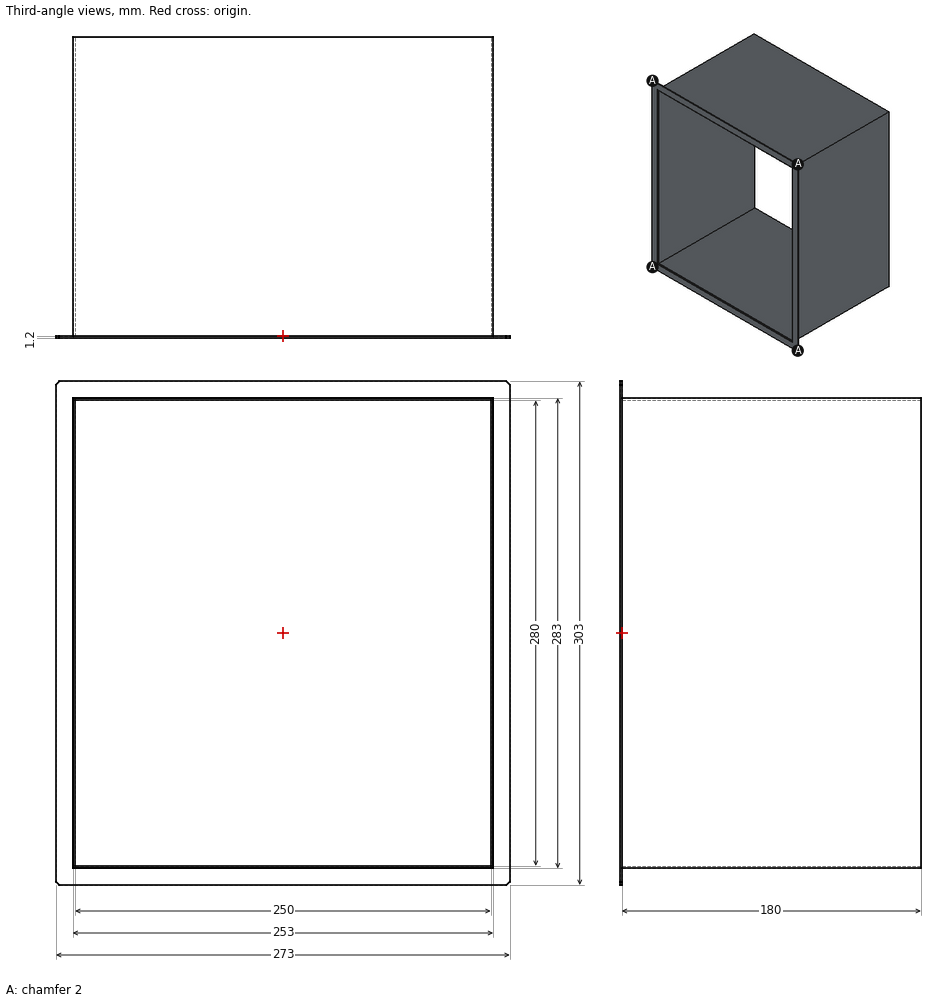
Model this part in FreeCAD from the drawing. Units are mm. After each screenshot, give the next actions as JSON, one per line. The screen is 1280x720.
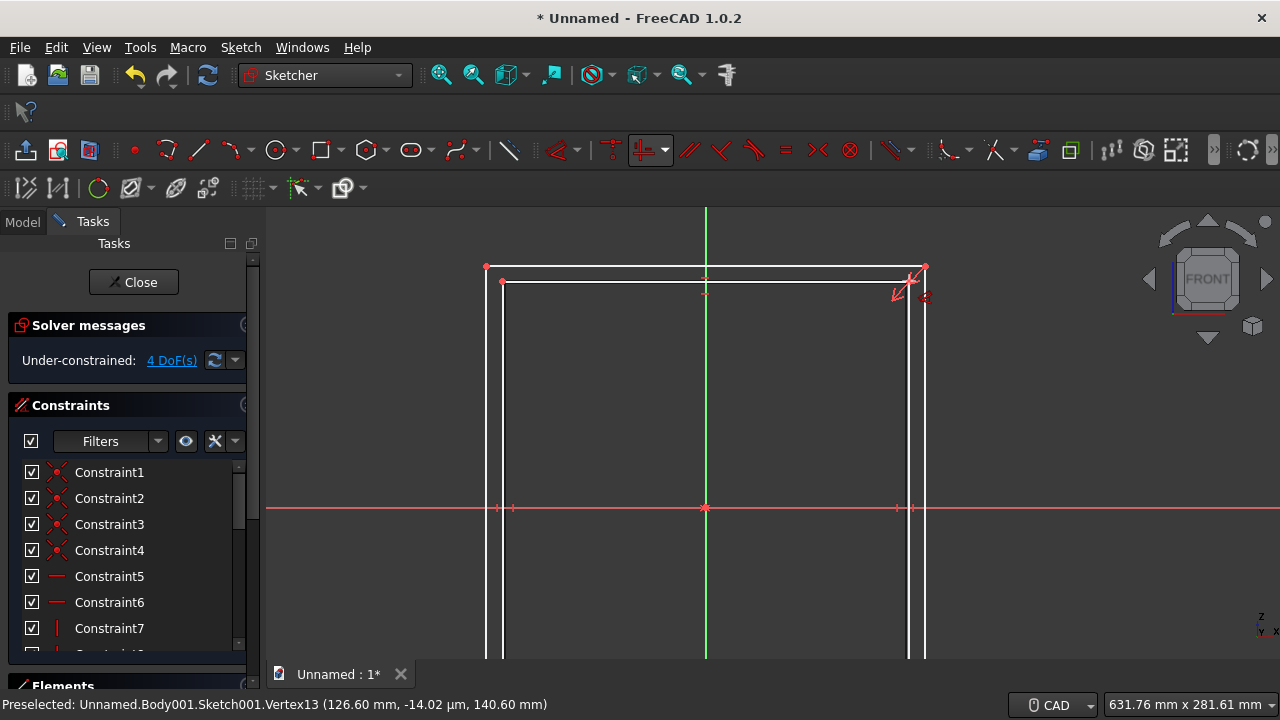
{"action": "scroll", "coordinate": [703, 342], "scroll_direction": "down", "scroll_amount": 3}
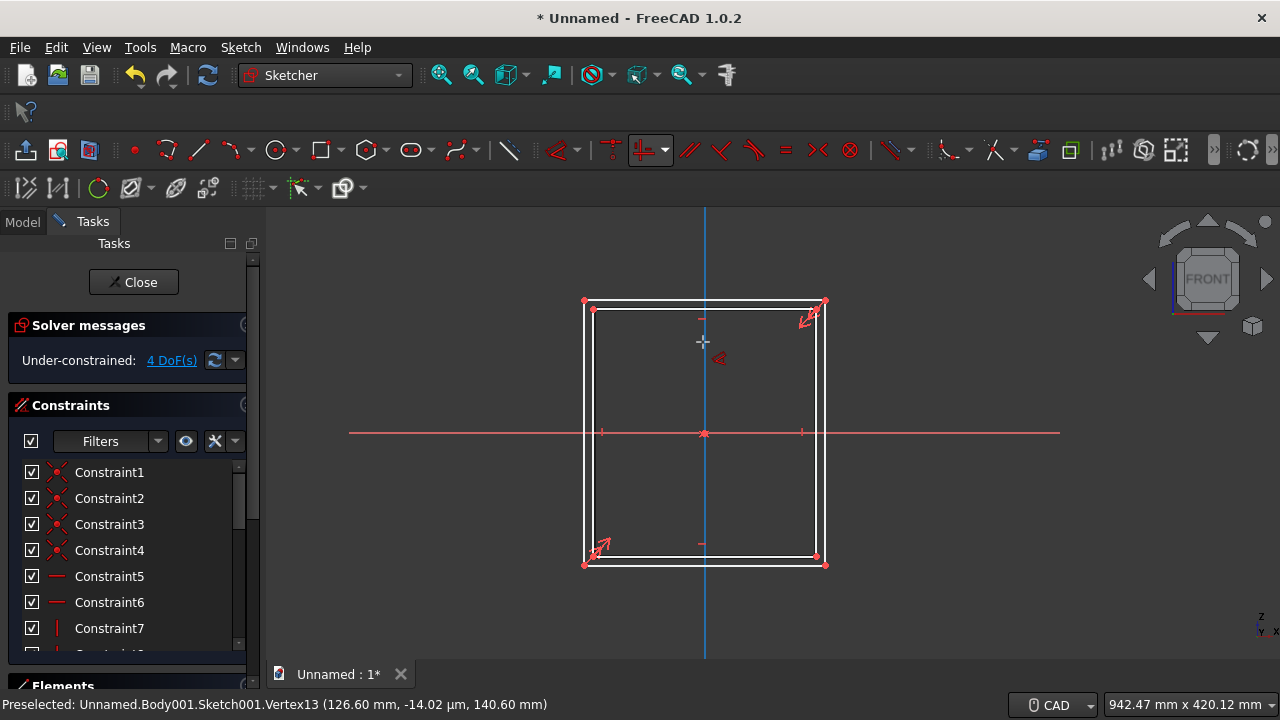
{"action": "scroll", "coordinate": [657, 566], "scroll_direction": "up", "scroll_amount": 3}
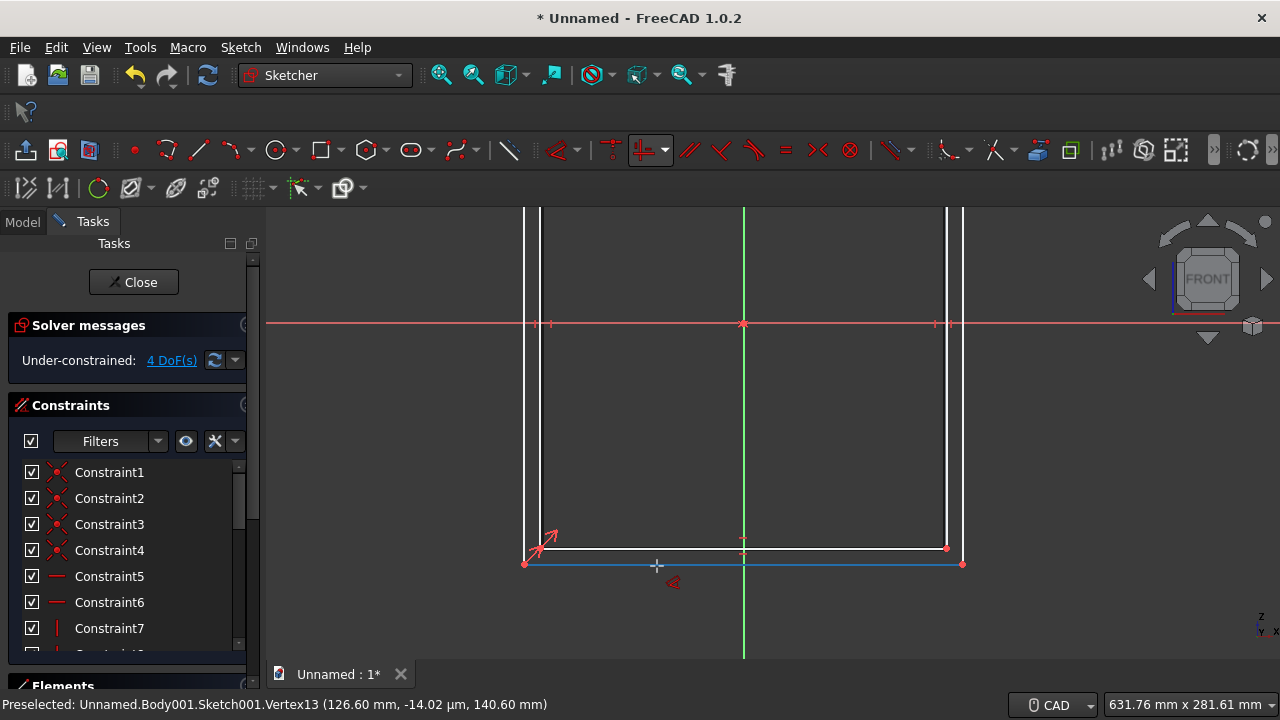
{"action": "left_click", "coordinate": [656, 565]}
{"action": "left_click", "coordinate": [643, 599]}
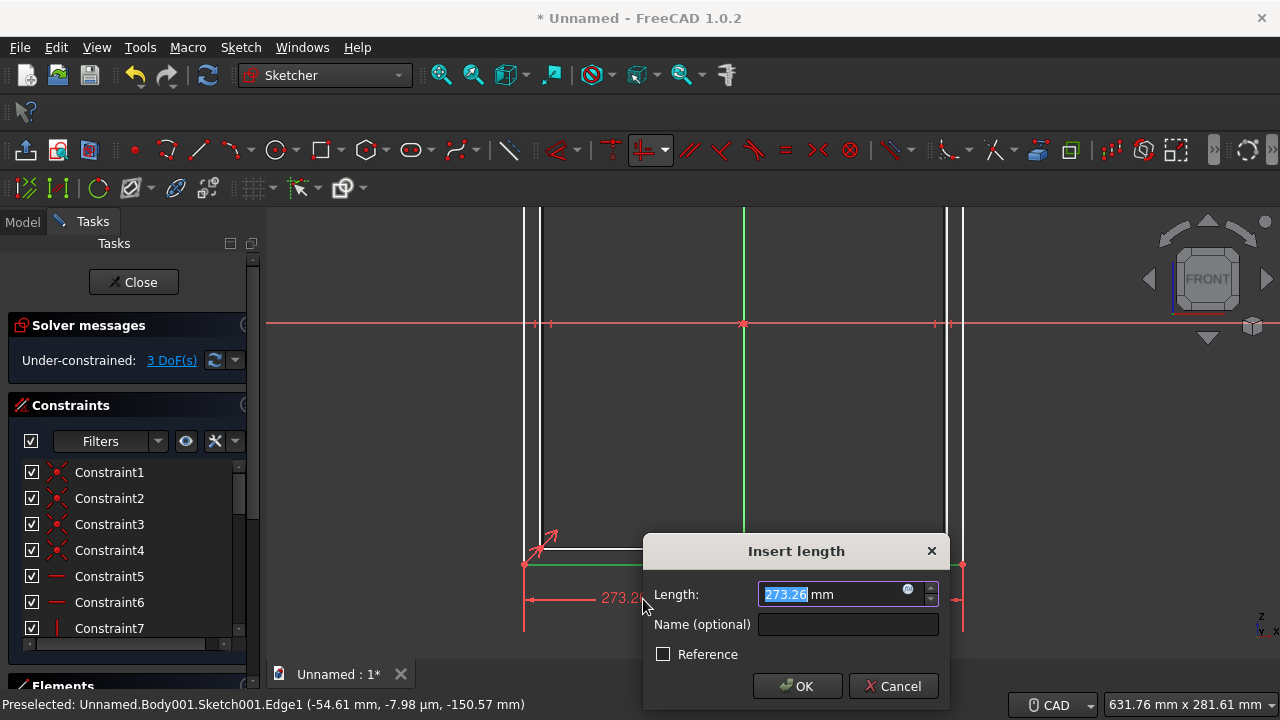
{"action": "type", "text": "273"}
{"action": "key", "text": "Return"}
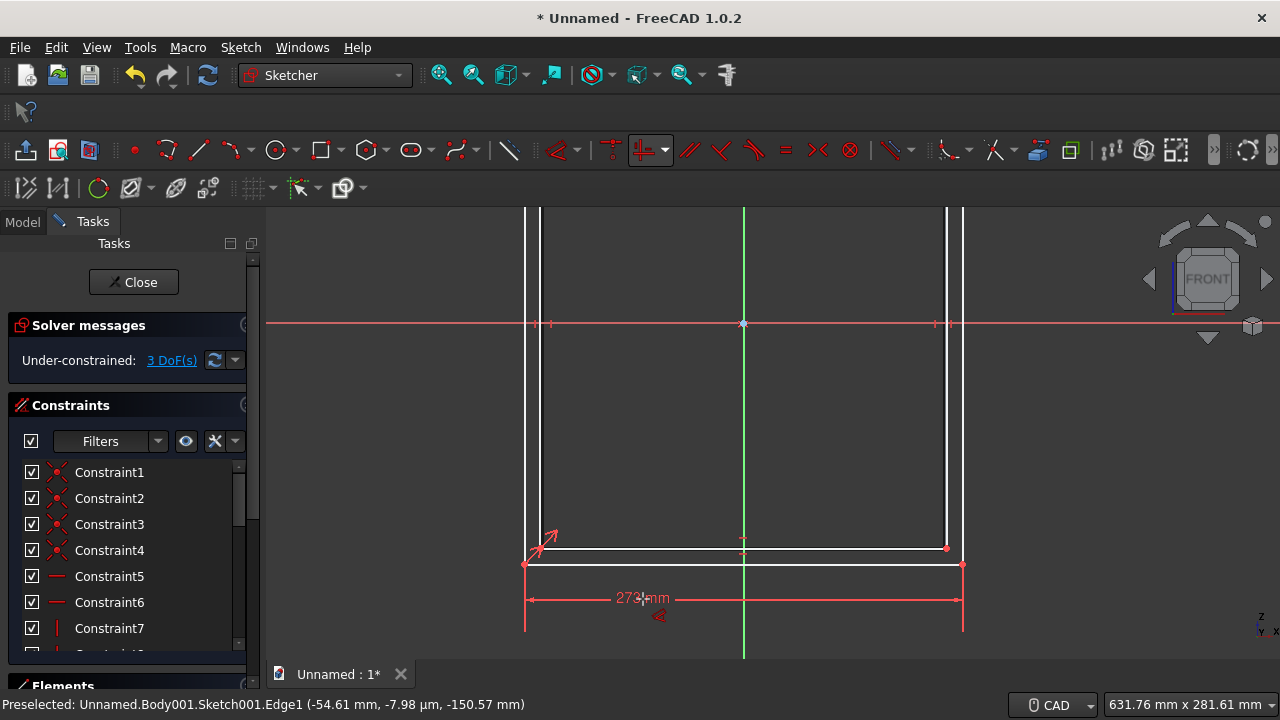
{"action": "left_click", "coordinate": [963, 420]}
{"action": "left_click", "coordinate": [997, 400]}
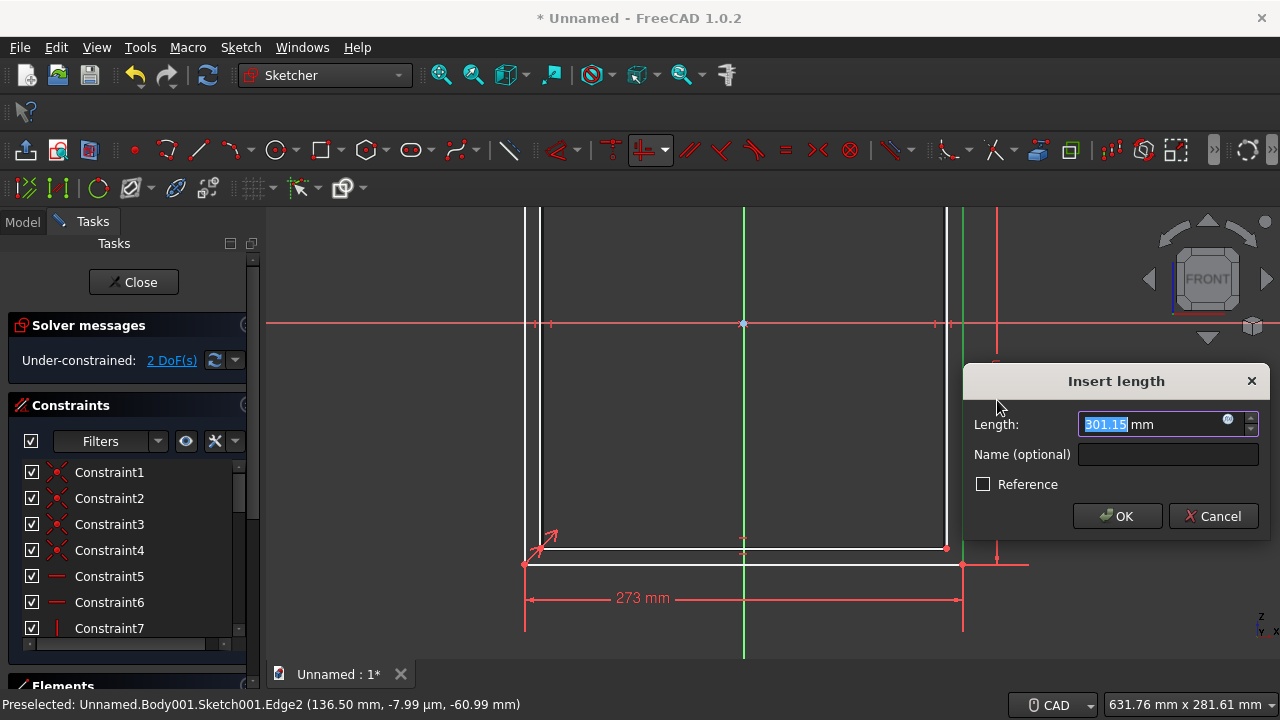
{"action": "type", "text": "303"}
{"action": "key", "text": "Return"}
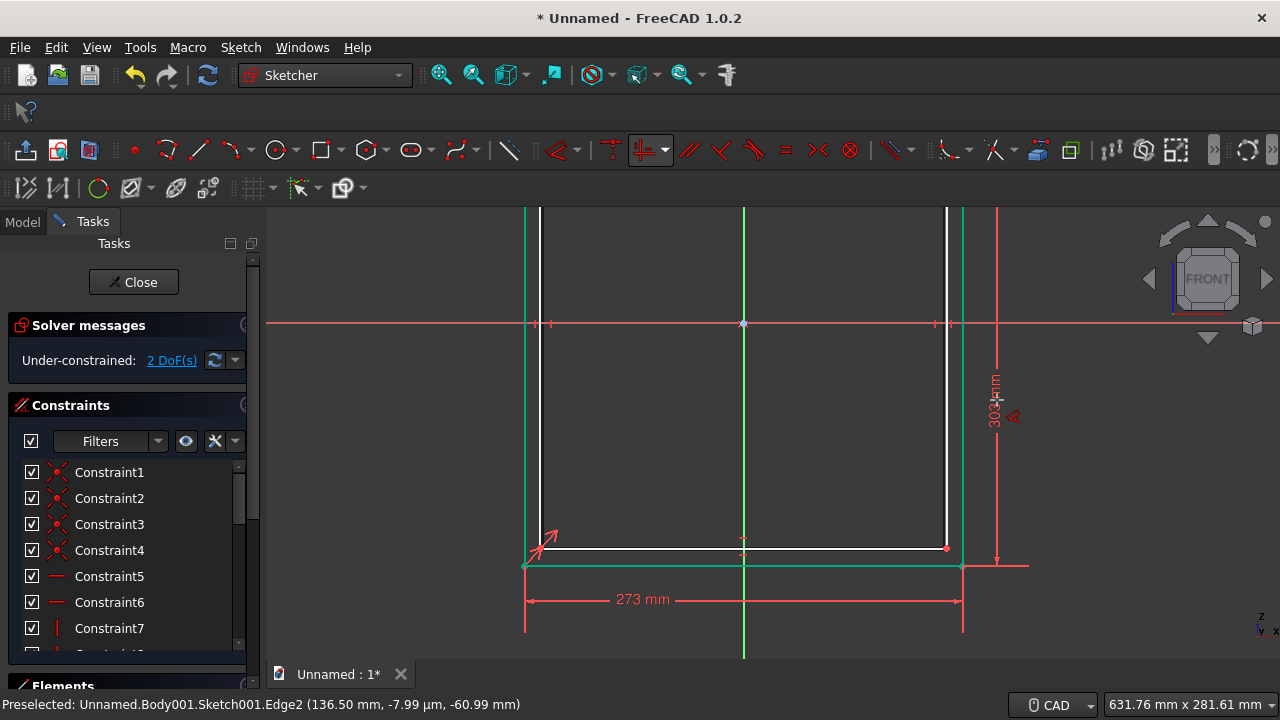
{"action": "left_click", "coordinate": [662, 549]}
{"action": "left_click", "coordinate": [837, 583]}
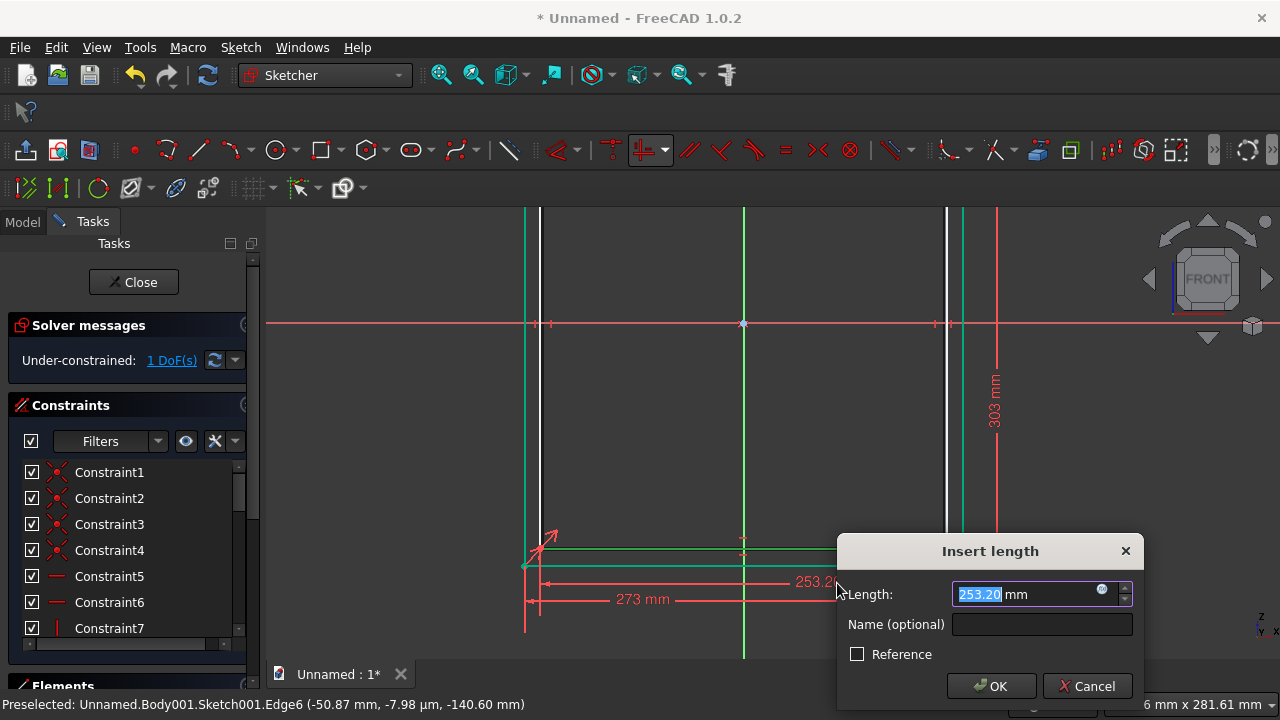
{"action": "type", "text": "253"}
{"action": "key", "text": "Return"}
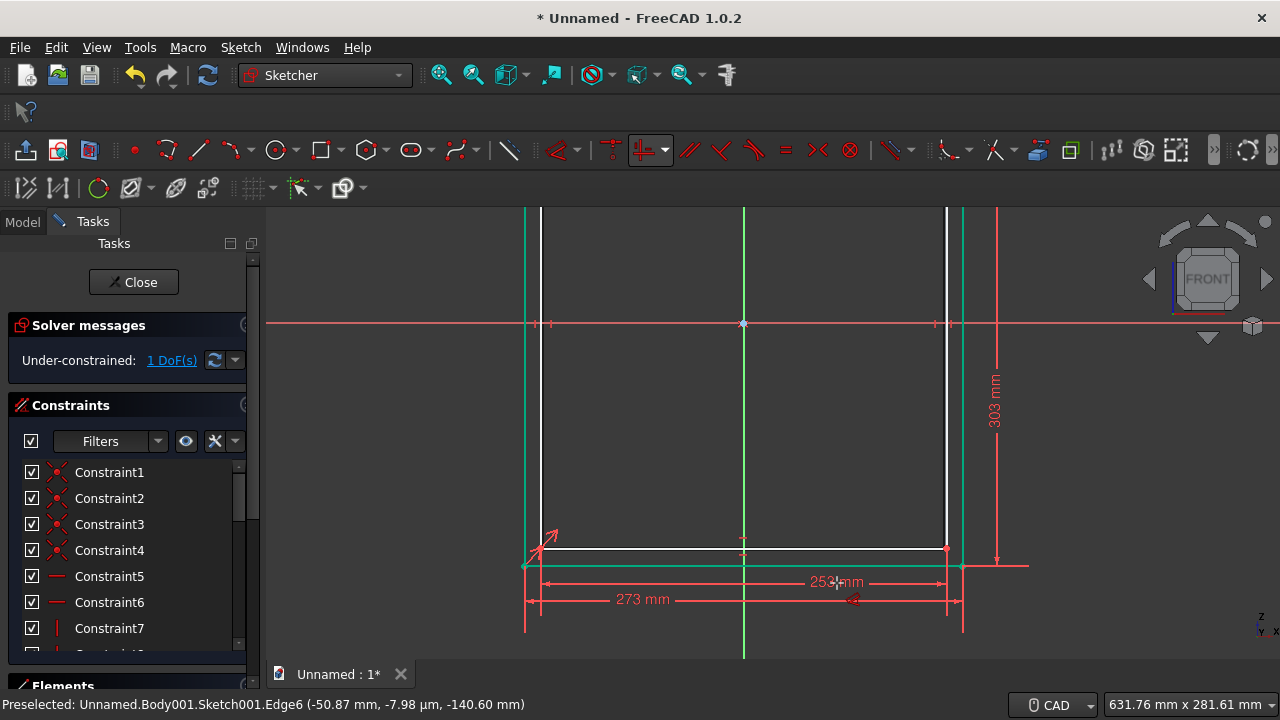
{"action": "left_click", "coordinate": [947, 413]}
{"action": "left_click", "coordinate": [981, 464]}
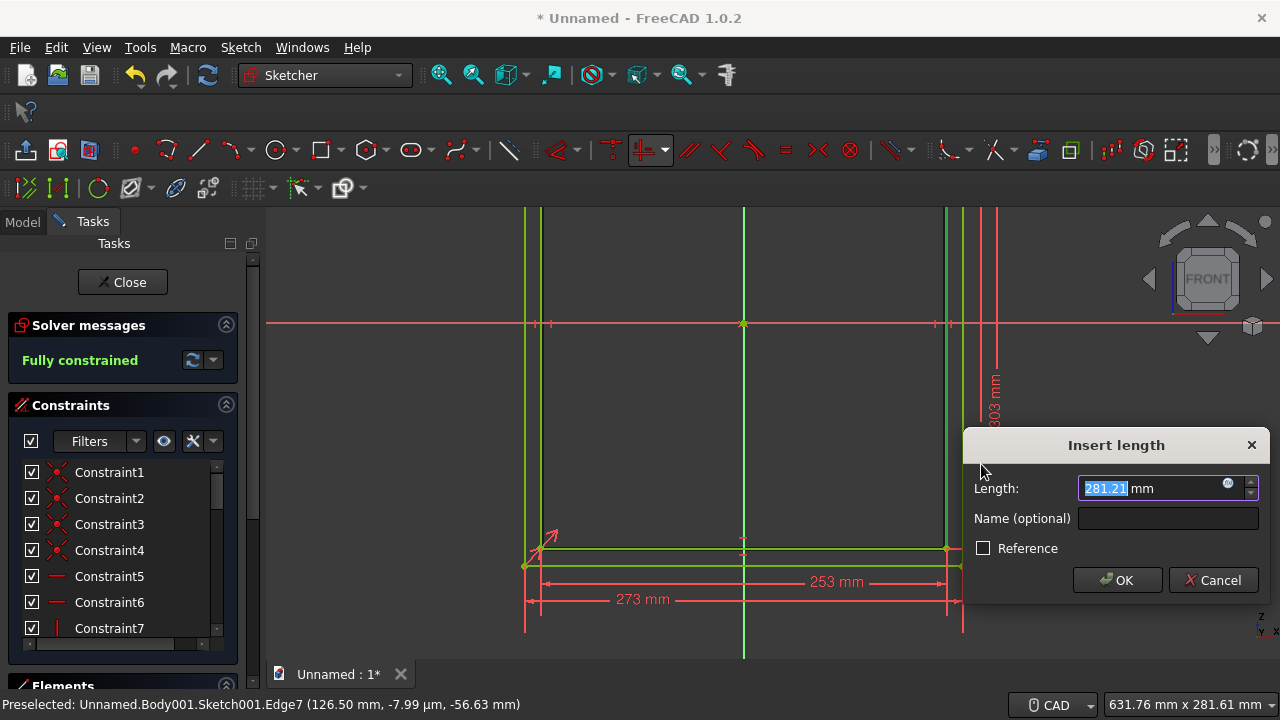
{"action": "type", "text": "283"}
{"action": "key", "text": "Return"}
{"action": "key", "text": "Escape"}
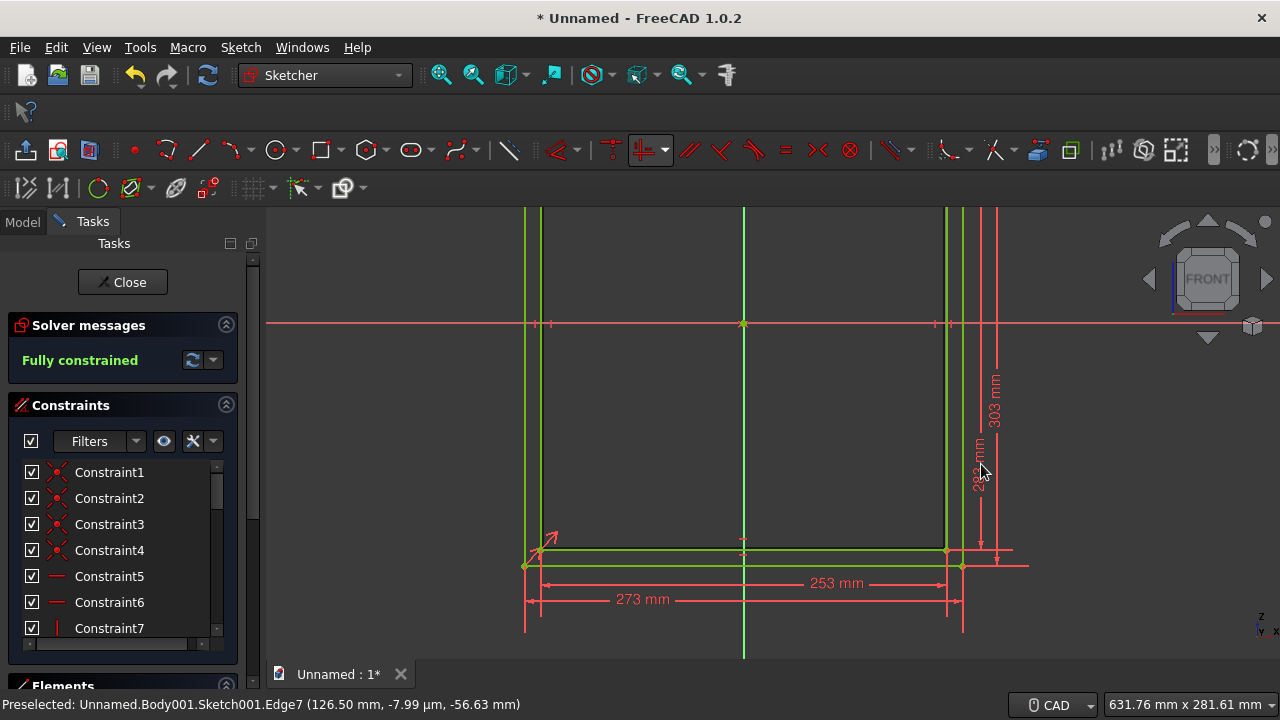
{"action": "left_click", "coordinate": [123, 282]}